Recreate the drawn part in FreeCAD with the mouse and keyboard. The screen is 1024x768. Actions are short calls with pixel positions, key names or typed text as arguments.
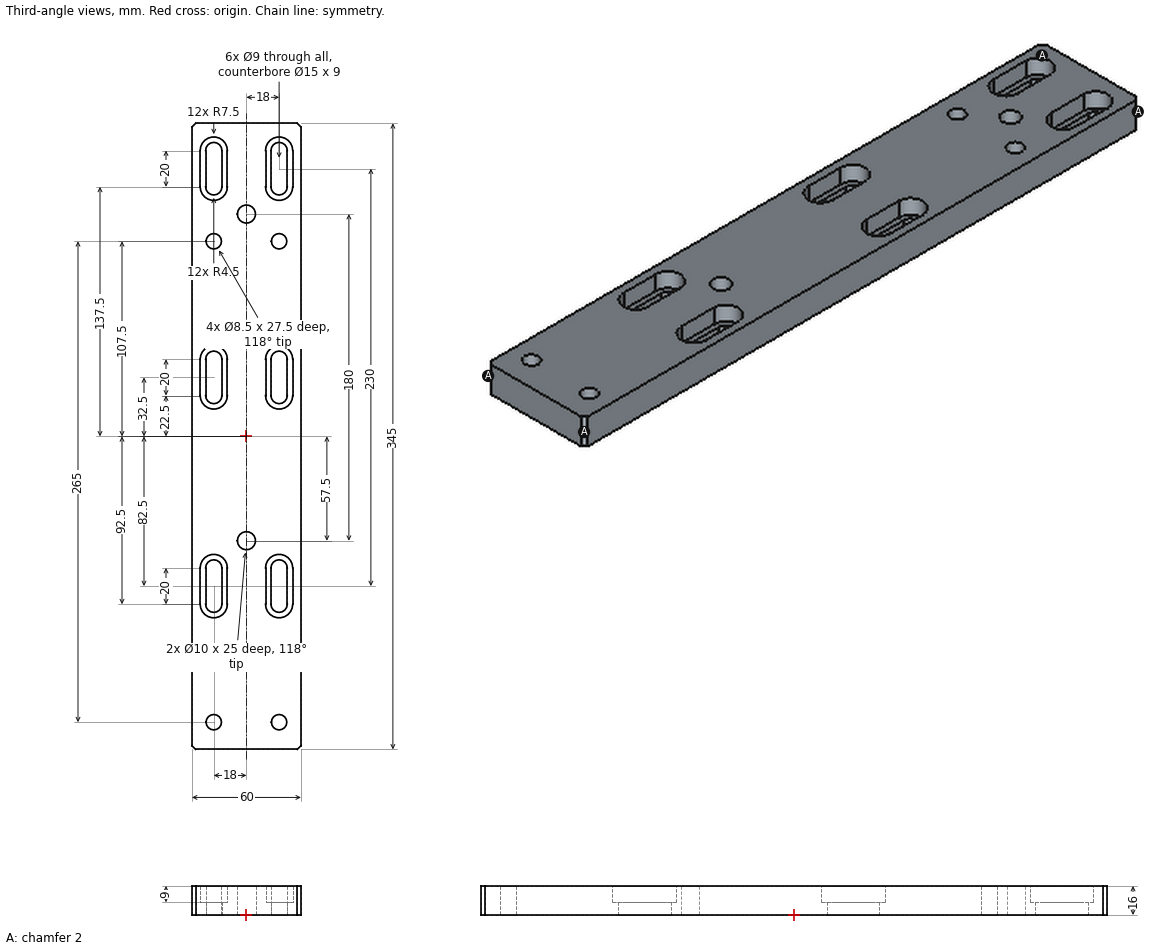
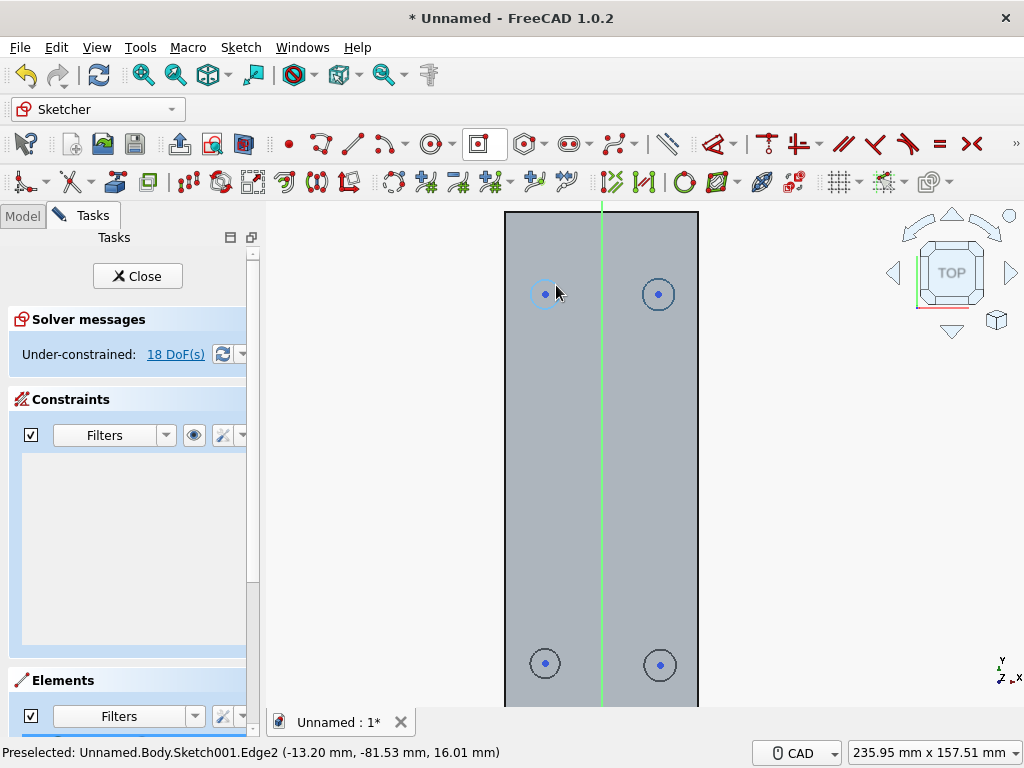
click(555, 284)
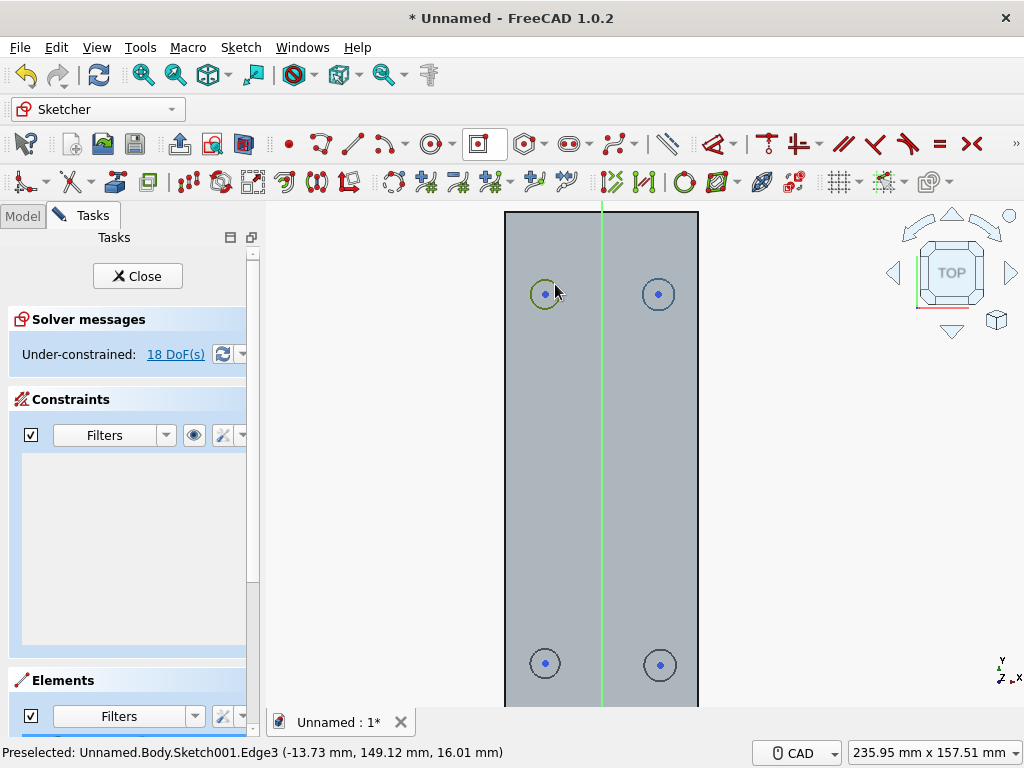
scroll(556, 284, down, 4)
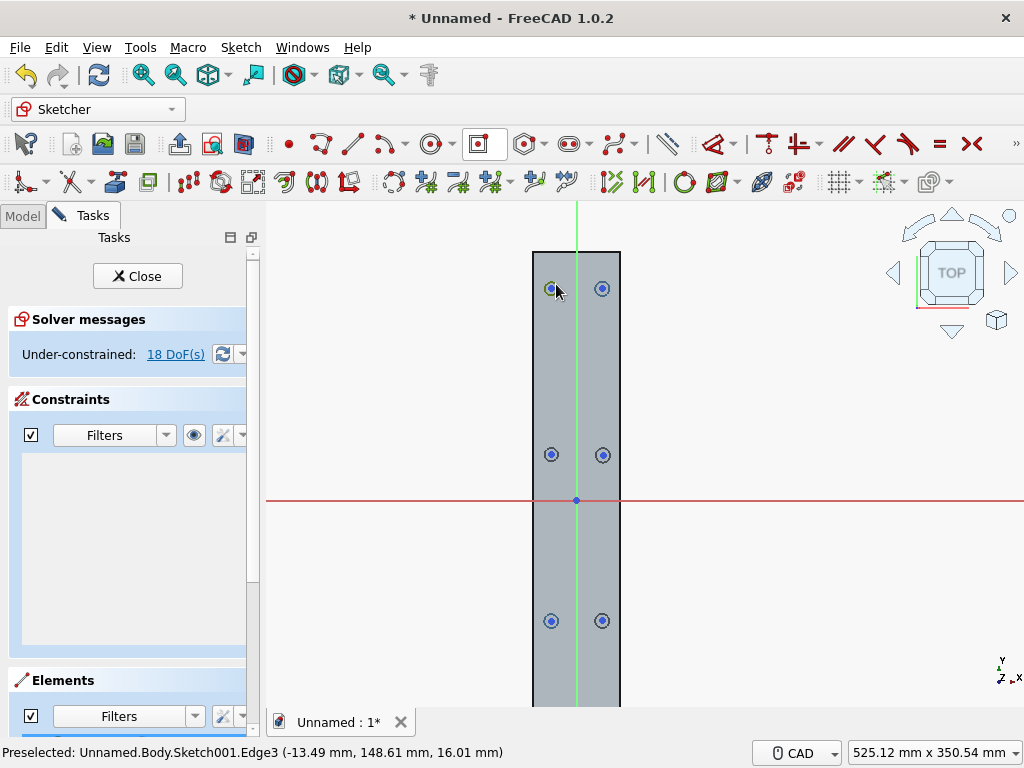
scroll(607, 616, up, 4)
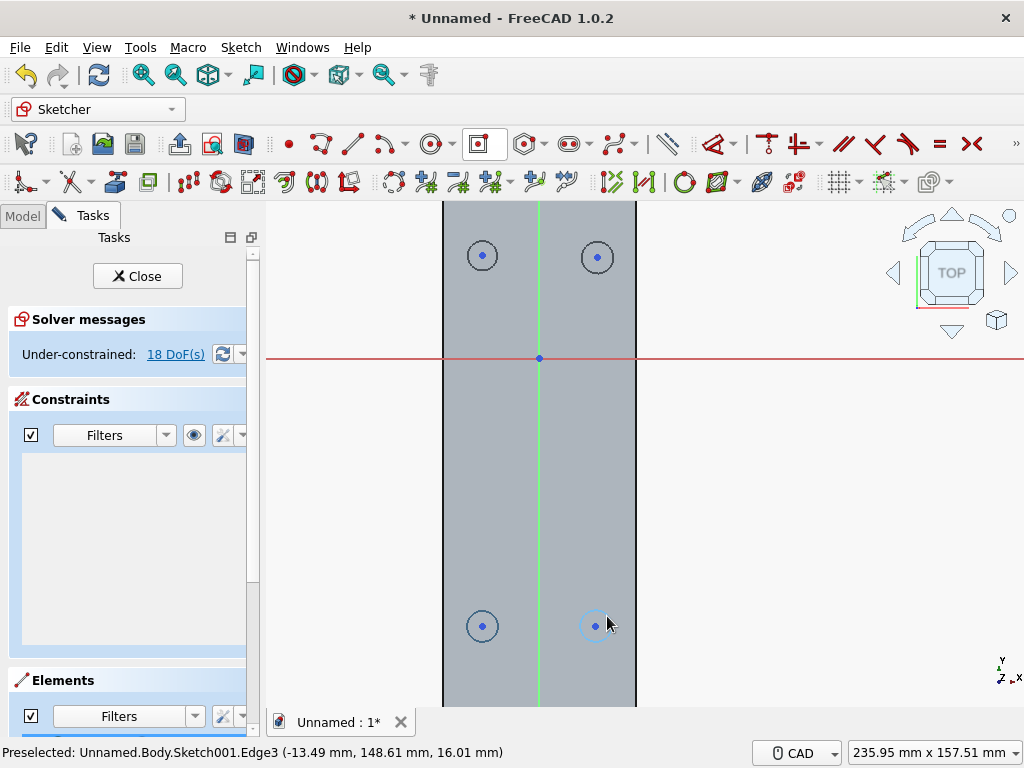
click(607, 615)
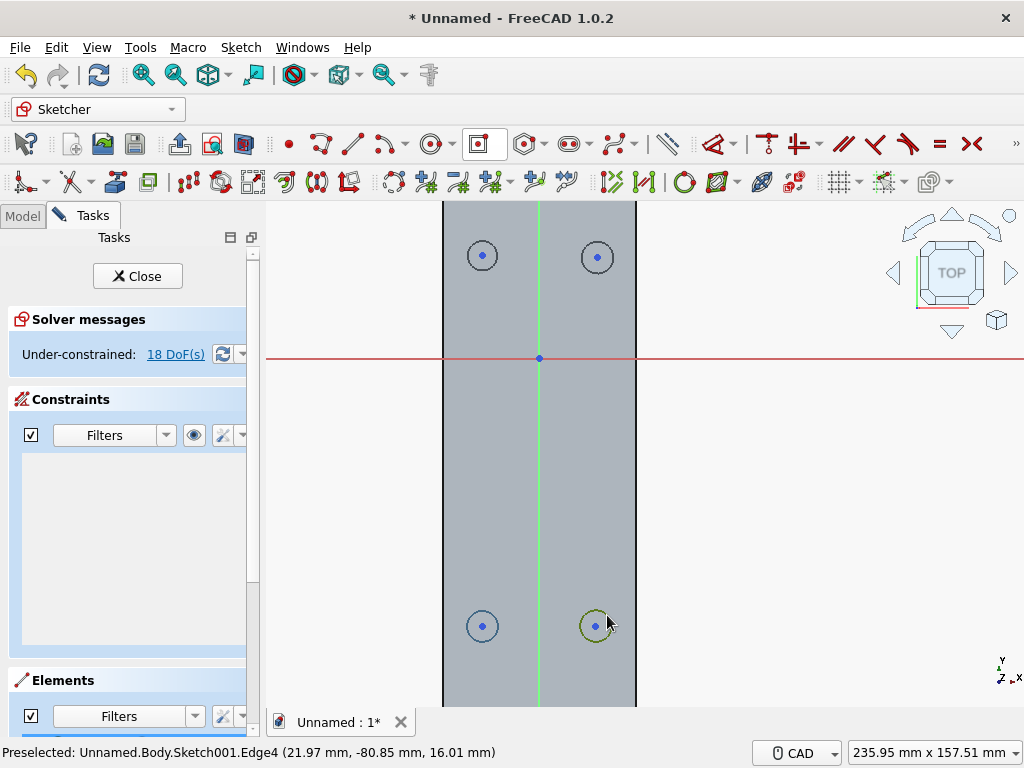
click(493, 245)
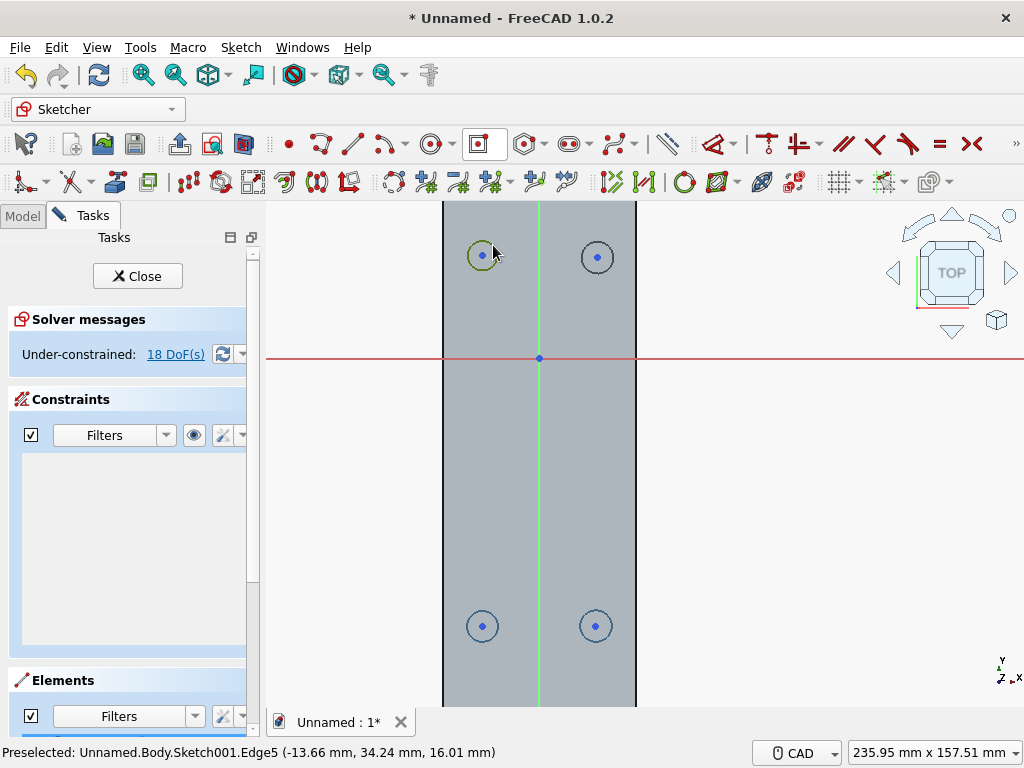
click(609, 246)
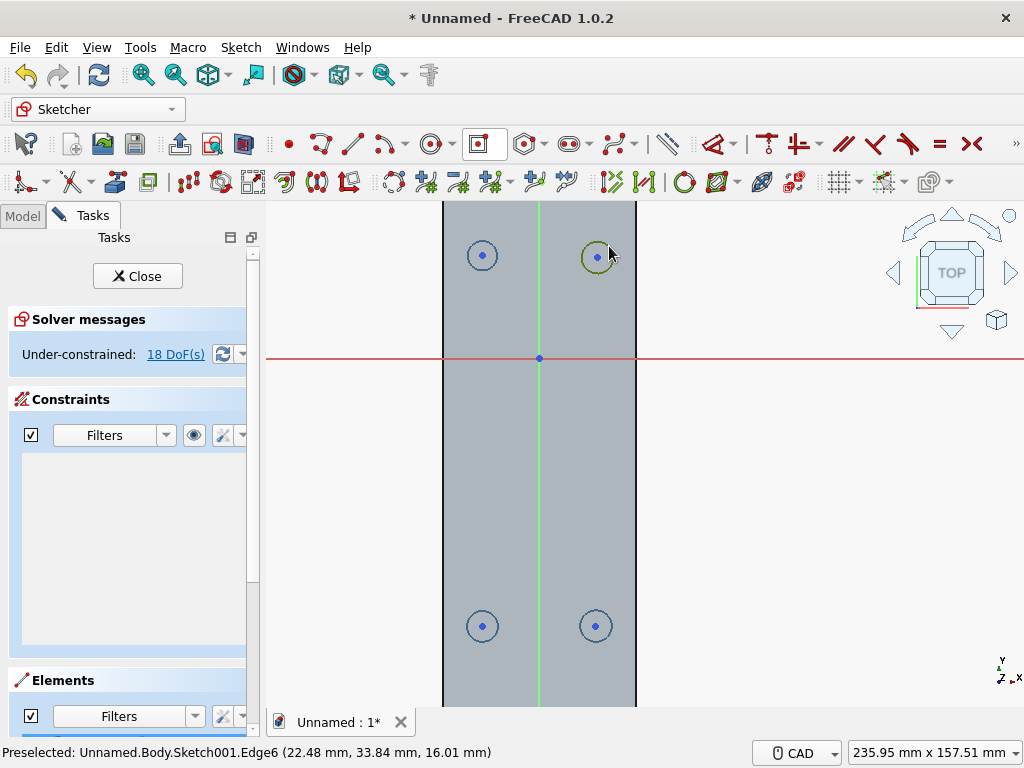
key(e)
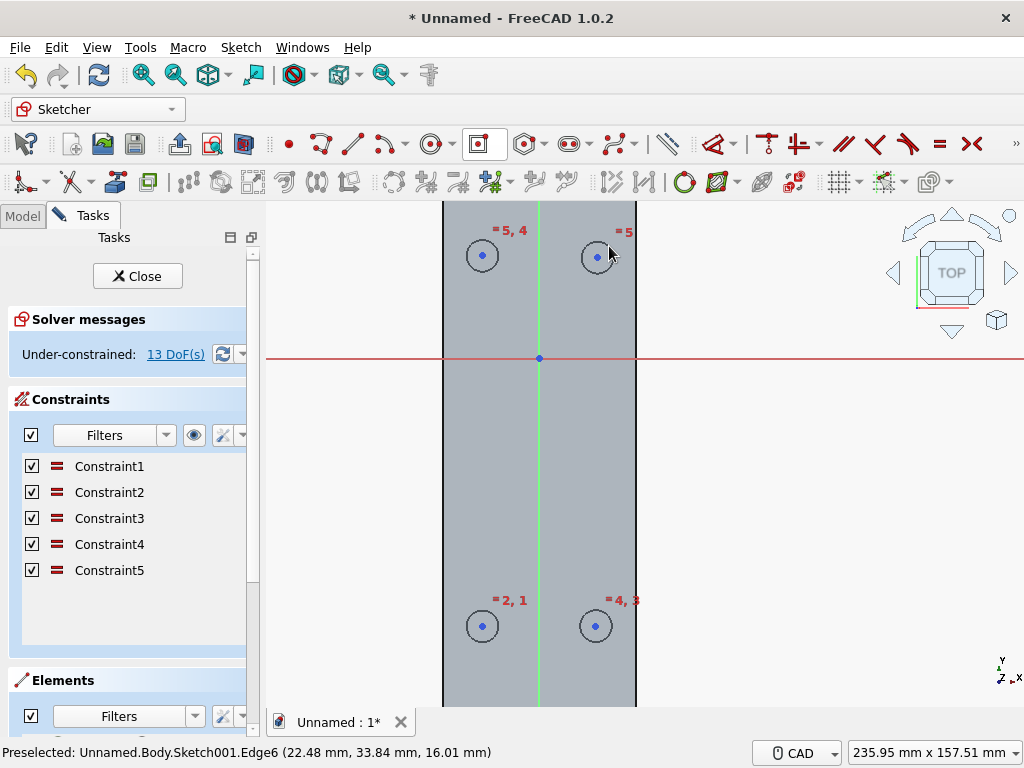
scroll(607, 617, down, 4)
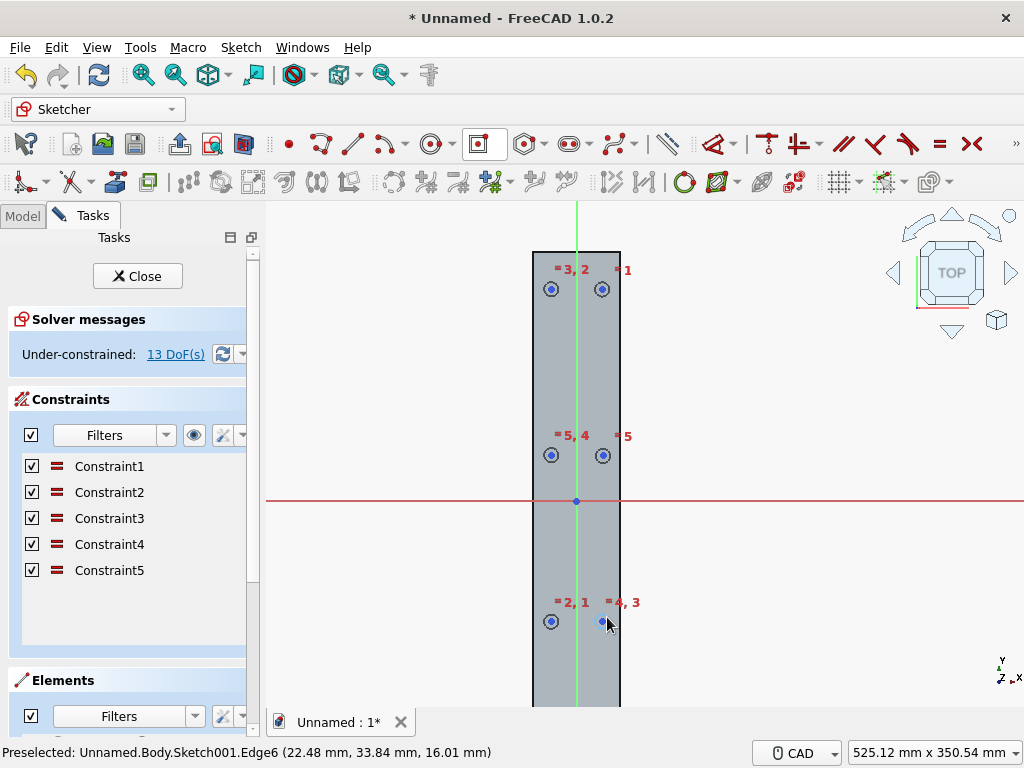
click(602, 289)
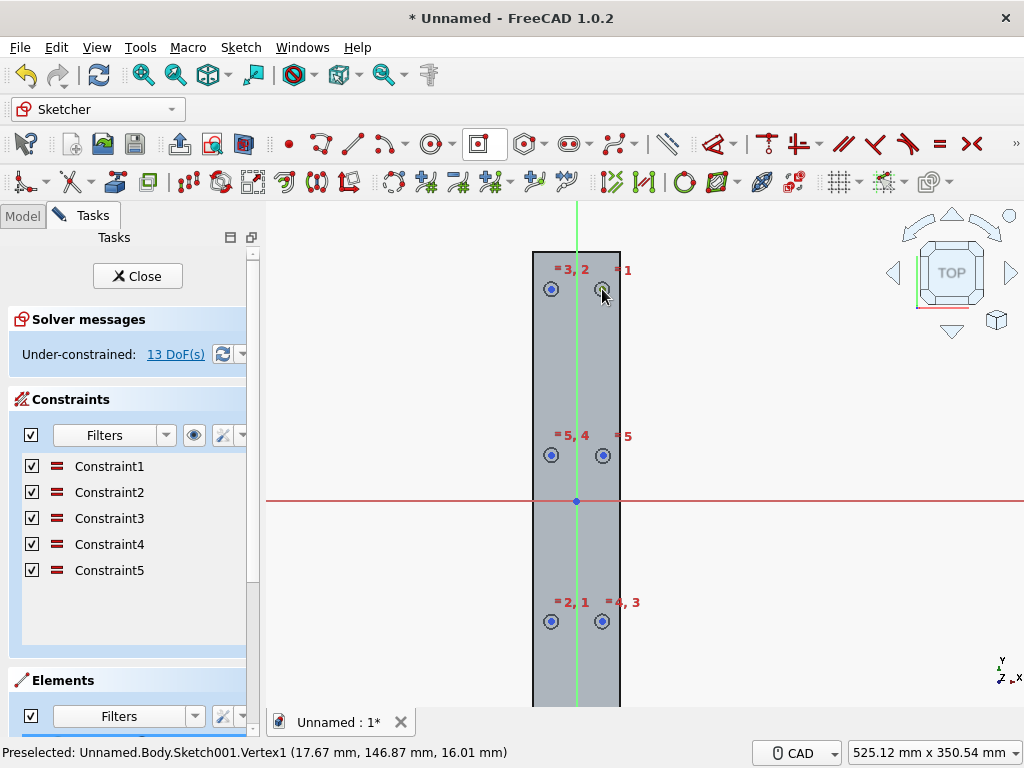
click(551, 289)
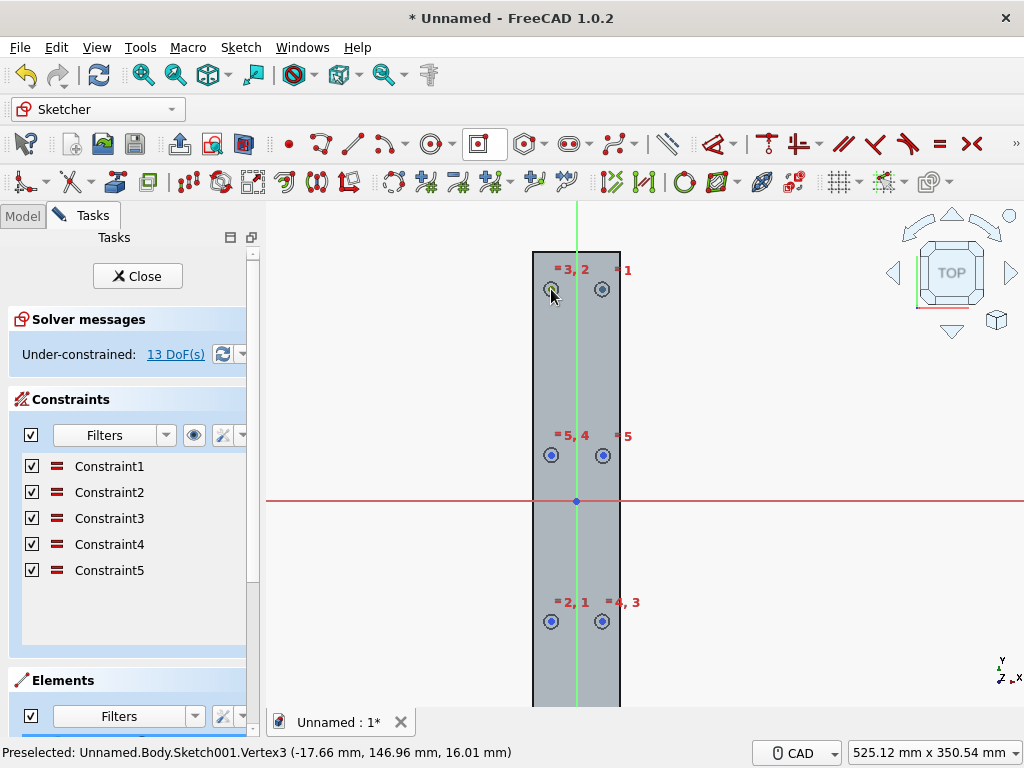
click(577, 583)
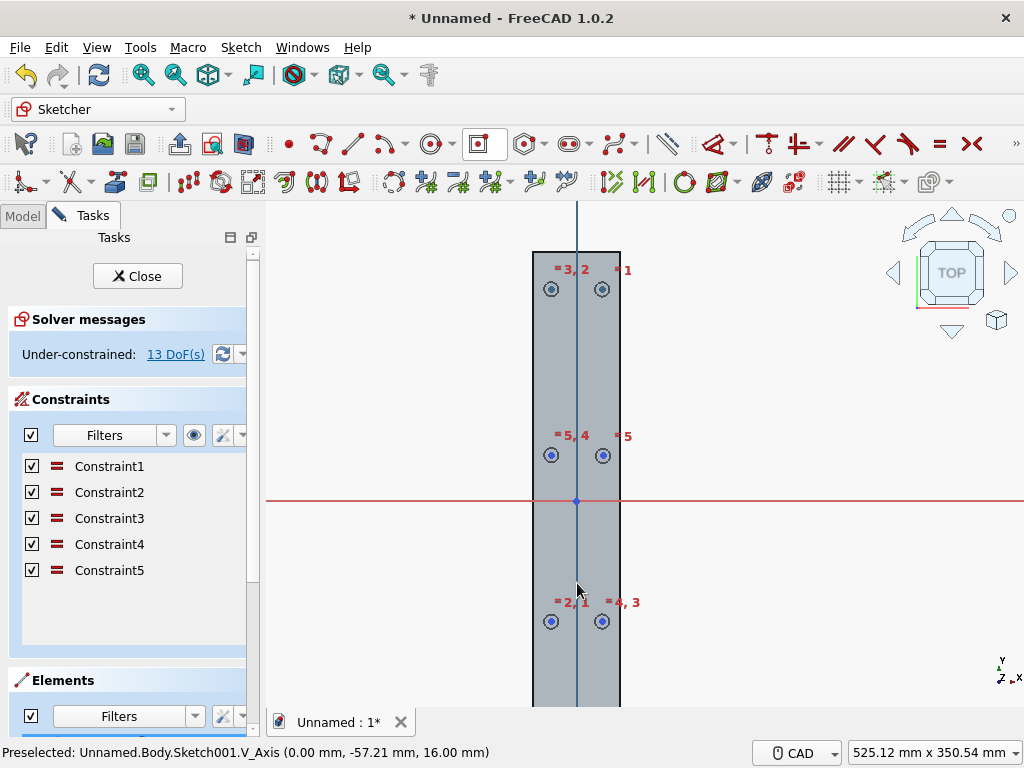
key(s)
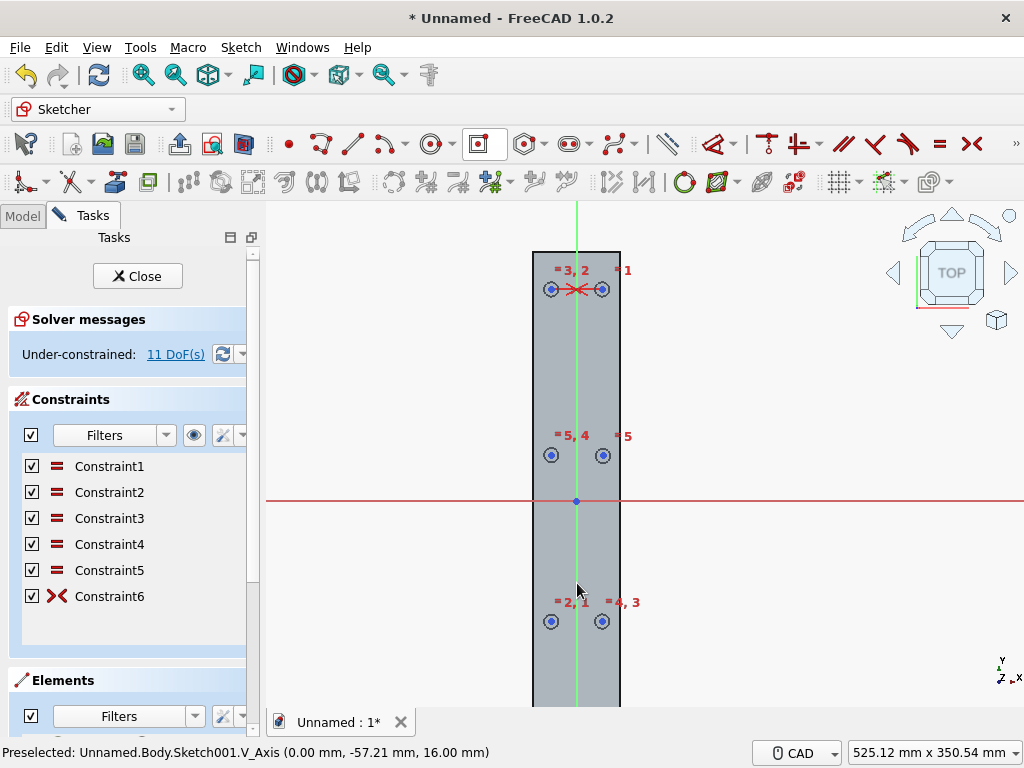
click(551, 622)